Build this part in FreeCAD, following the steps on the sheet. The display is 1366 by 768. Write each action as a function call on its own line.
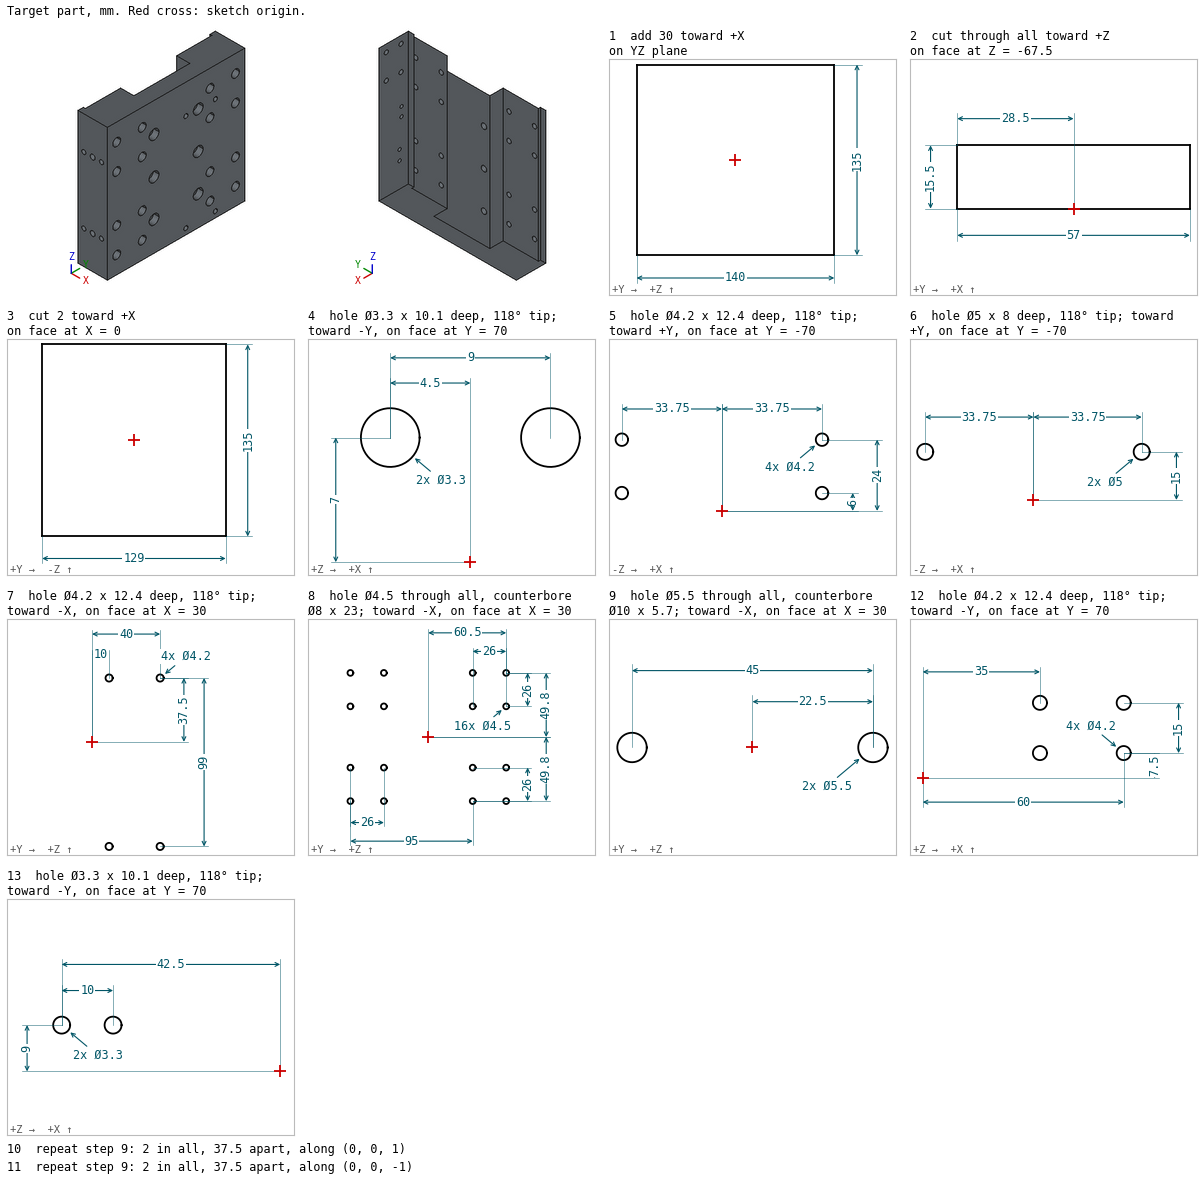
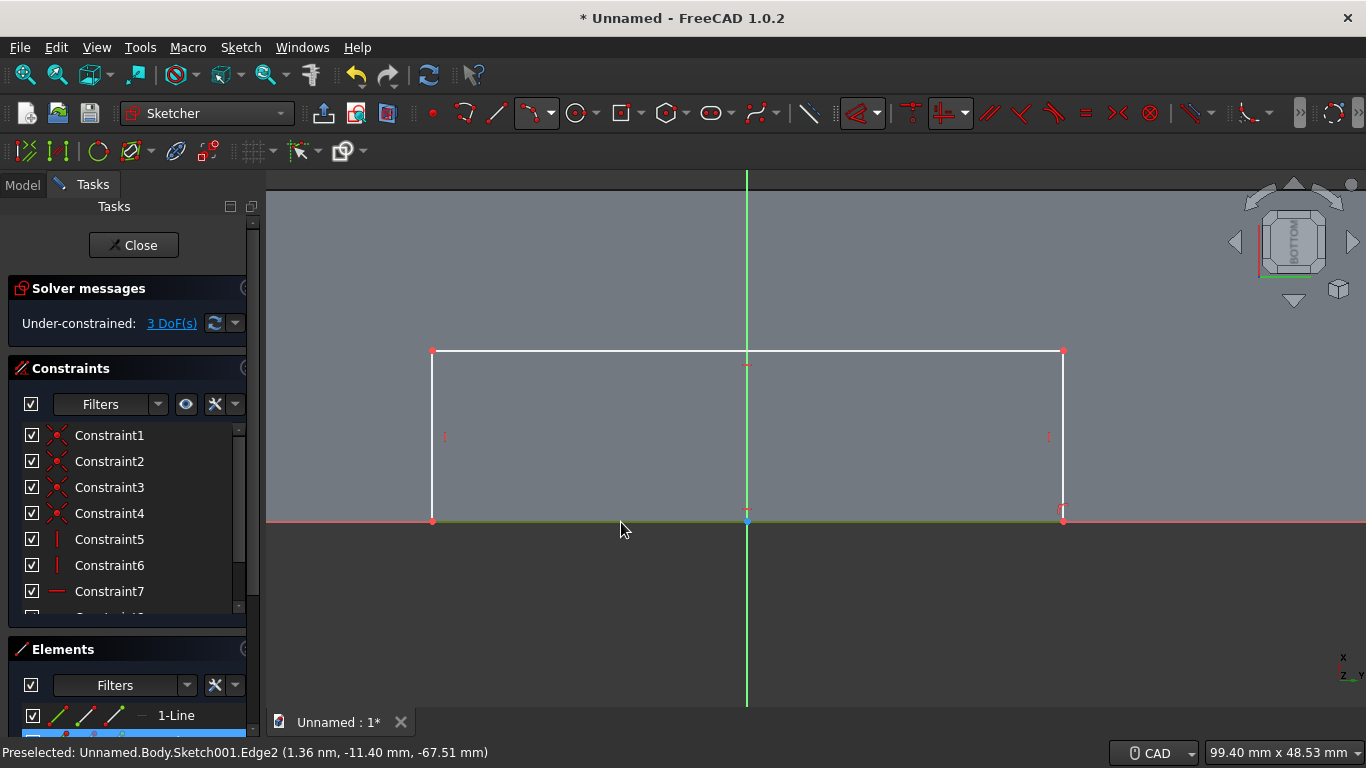
key(l)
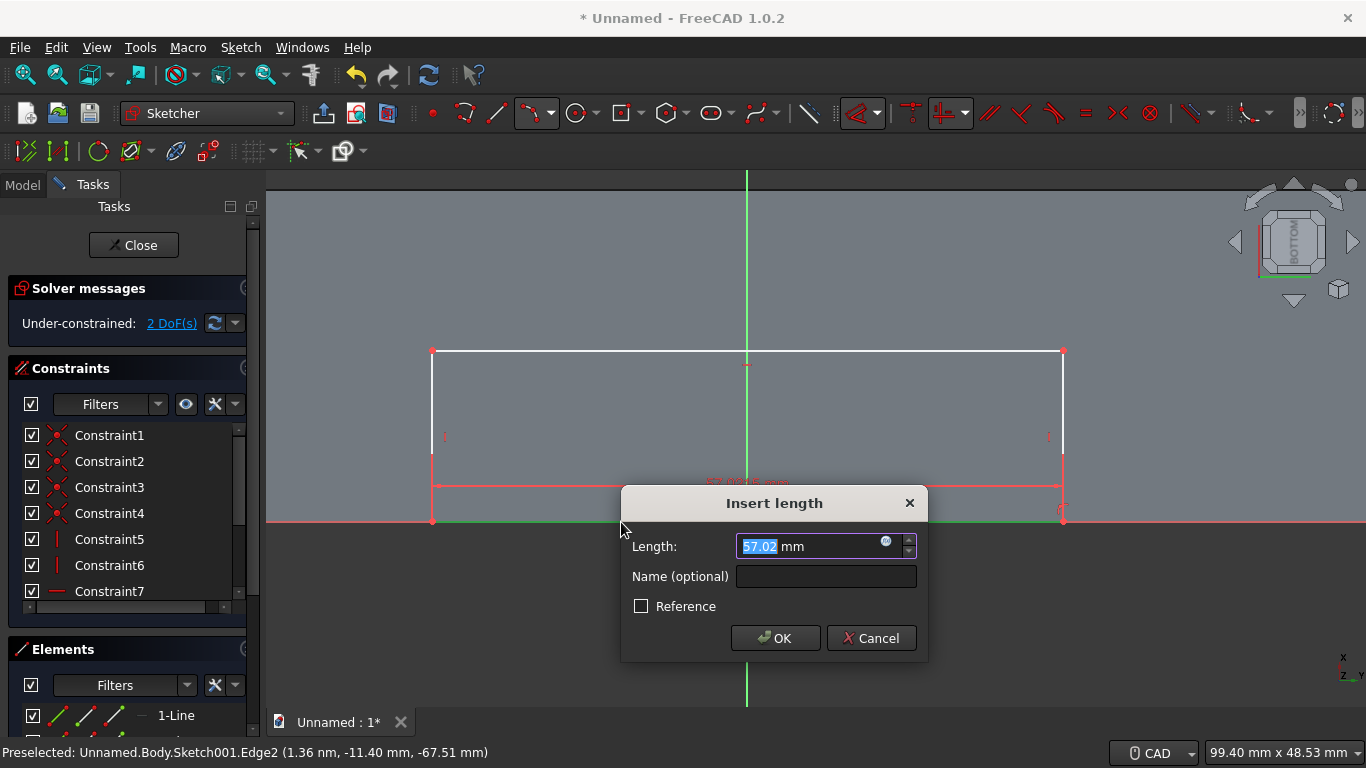
text(57)
key(Return)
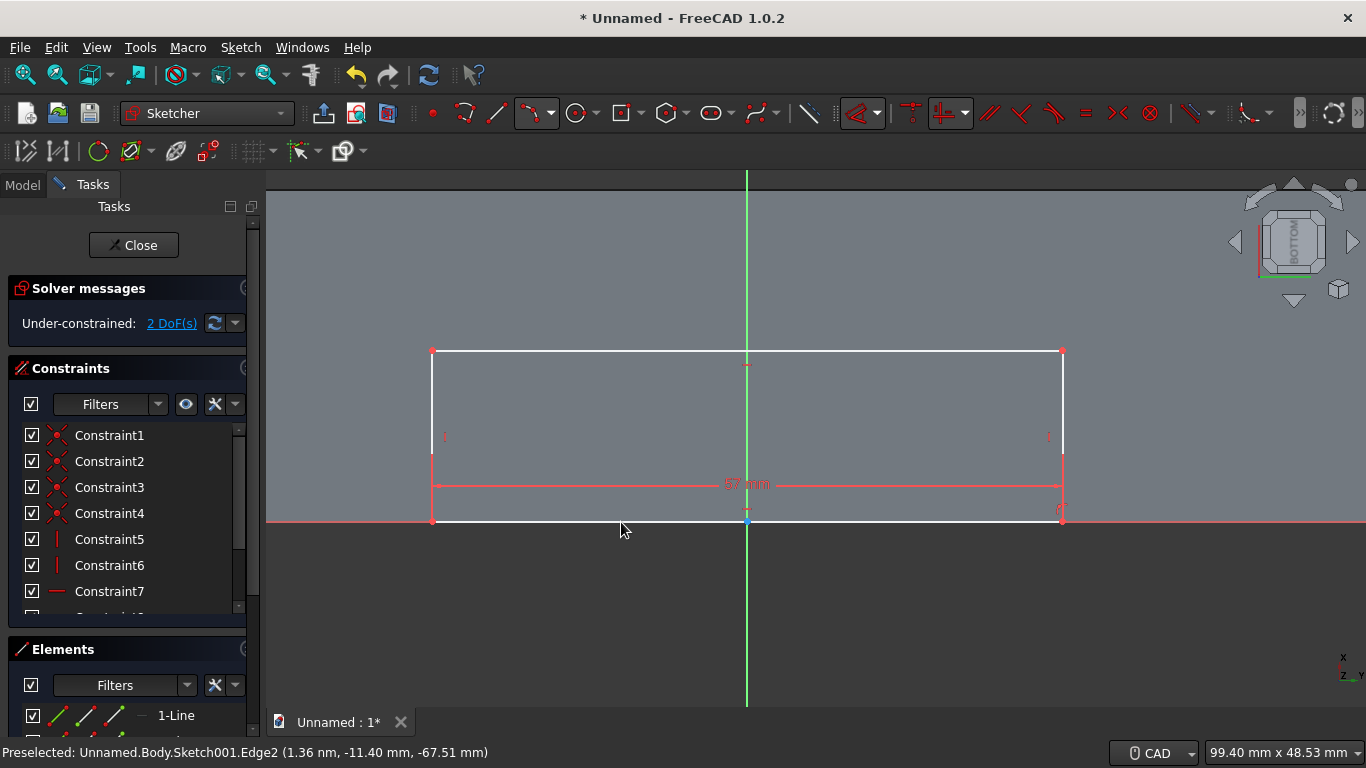
click(432, 402)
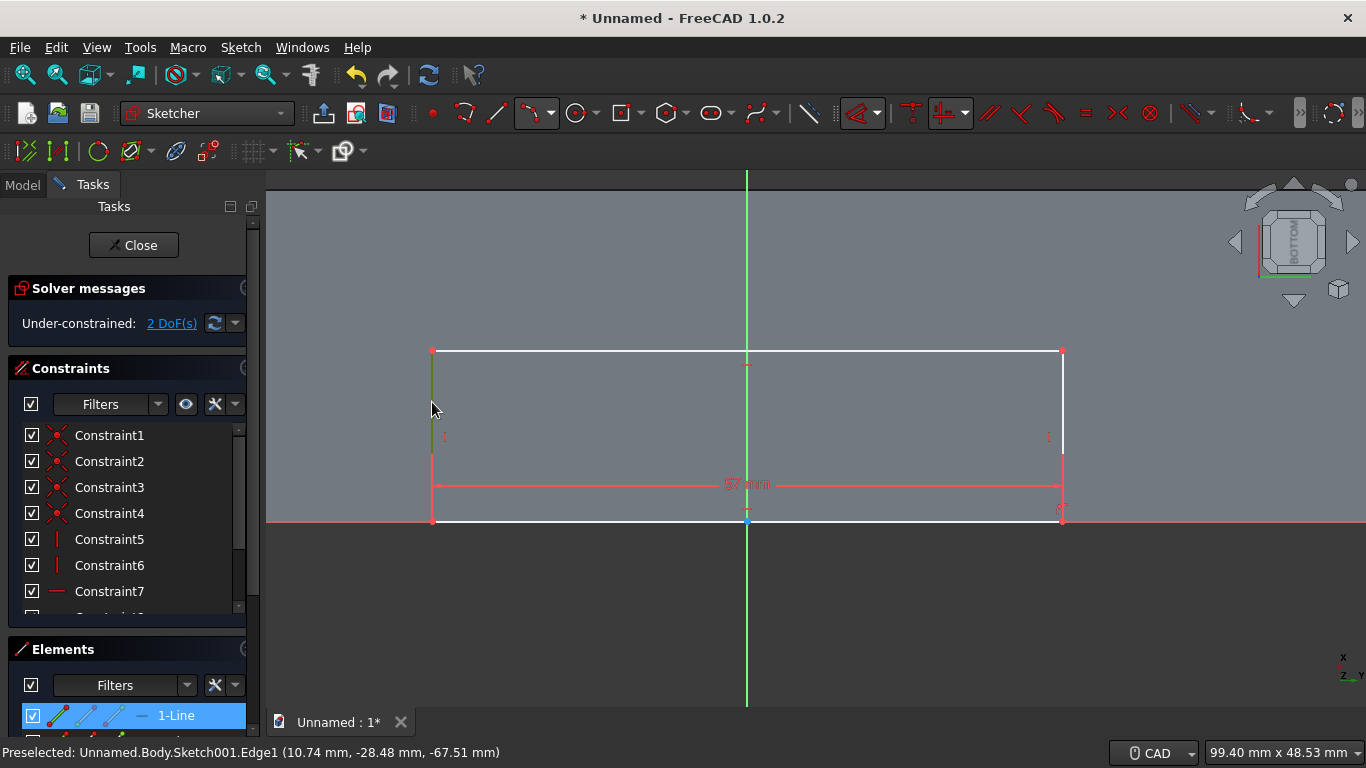
click(880, 114)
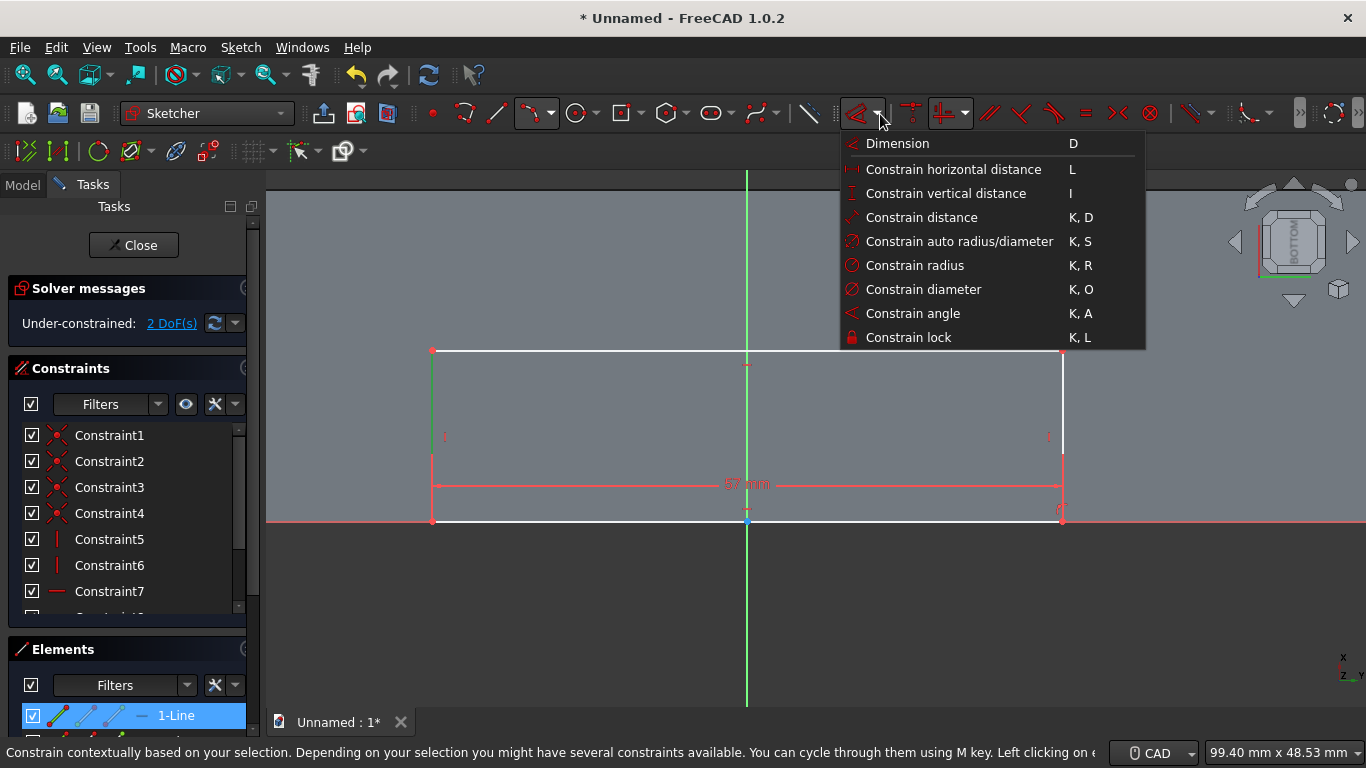
click(993, 193)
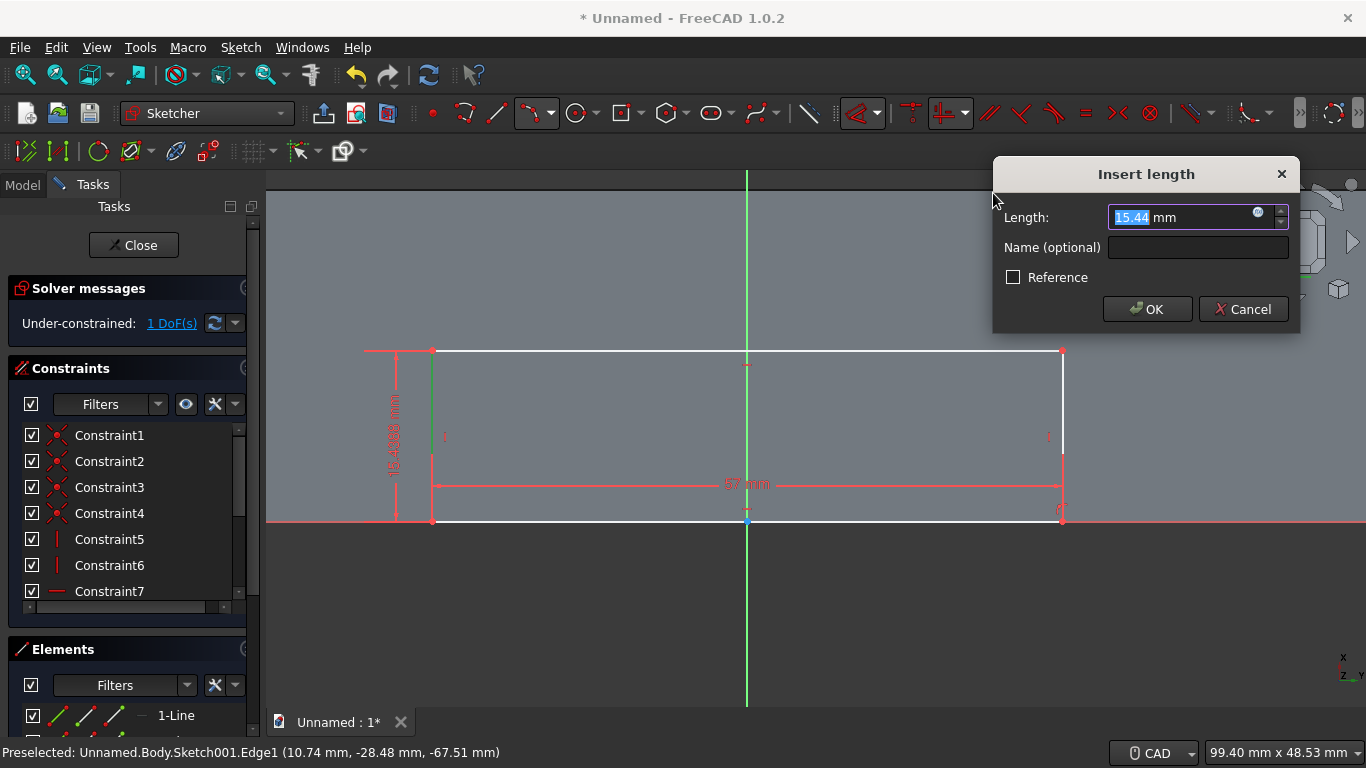
text(15.5)
key(Return)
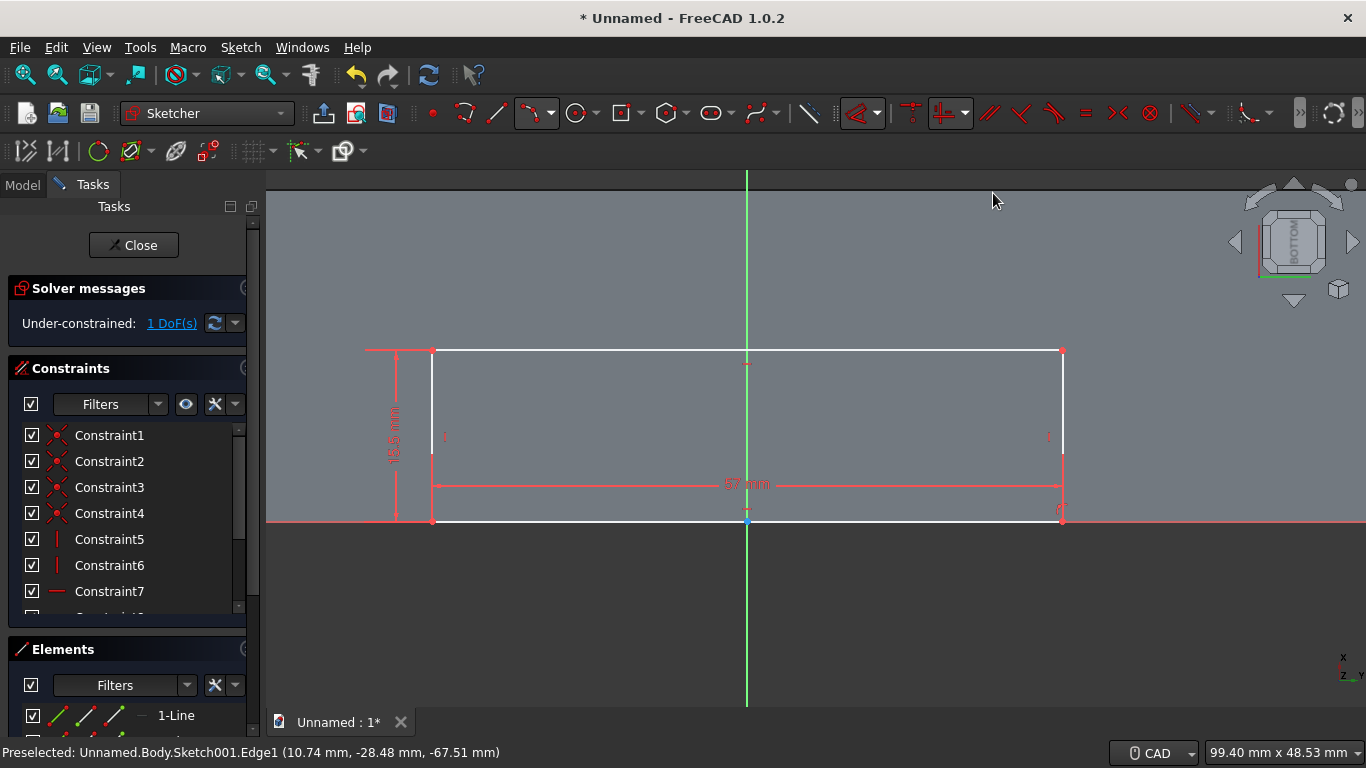
click(432, 350)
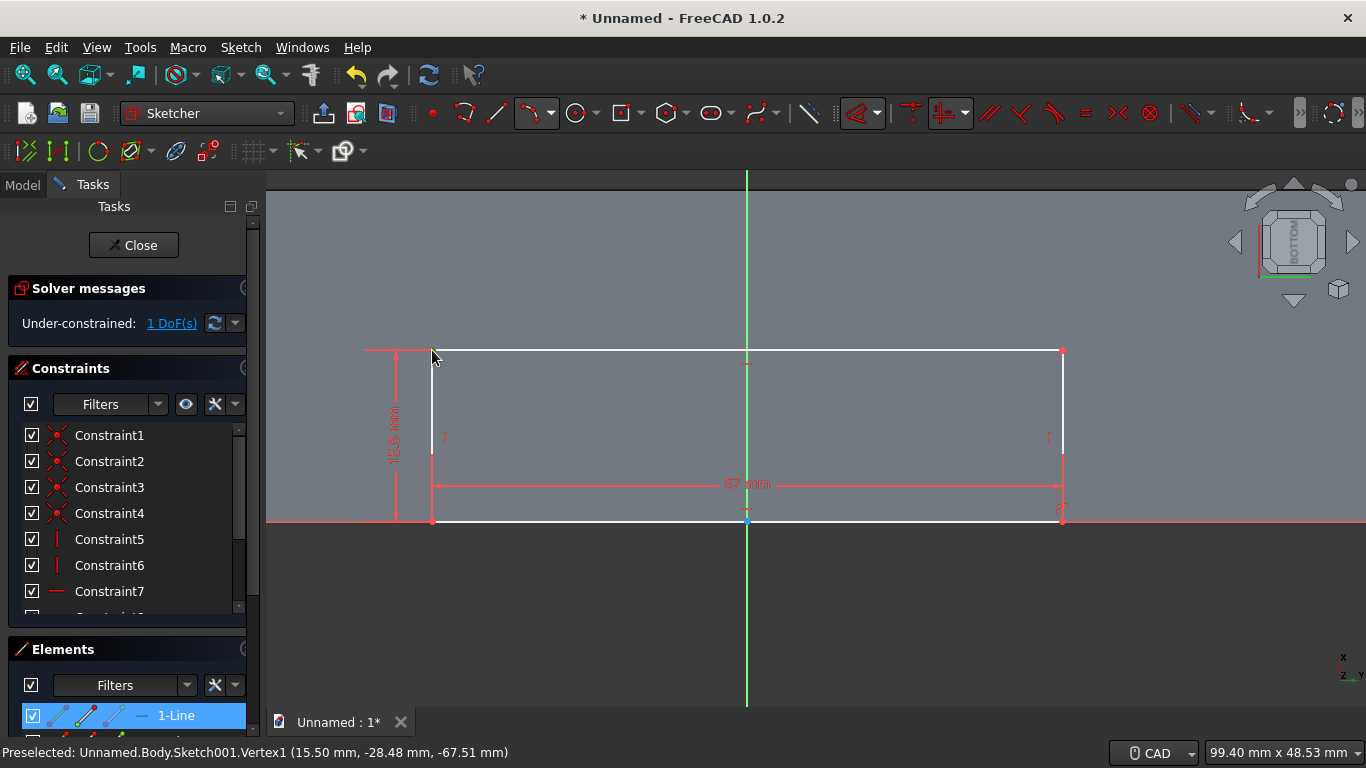
click(880, 114)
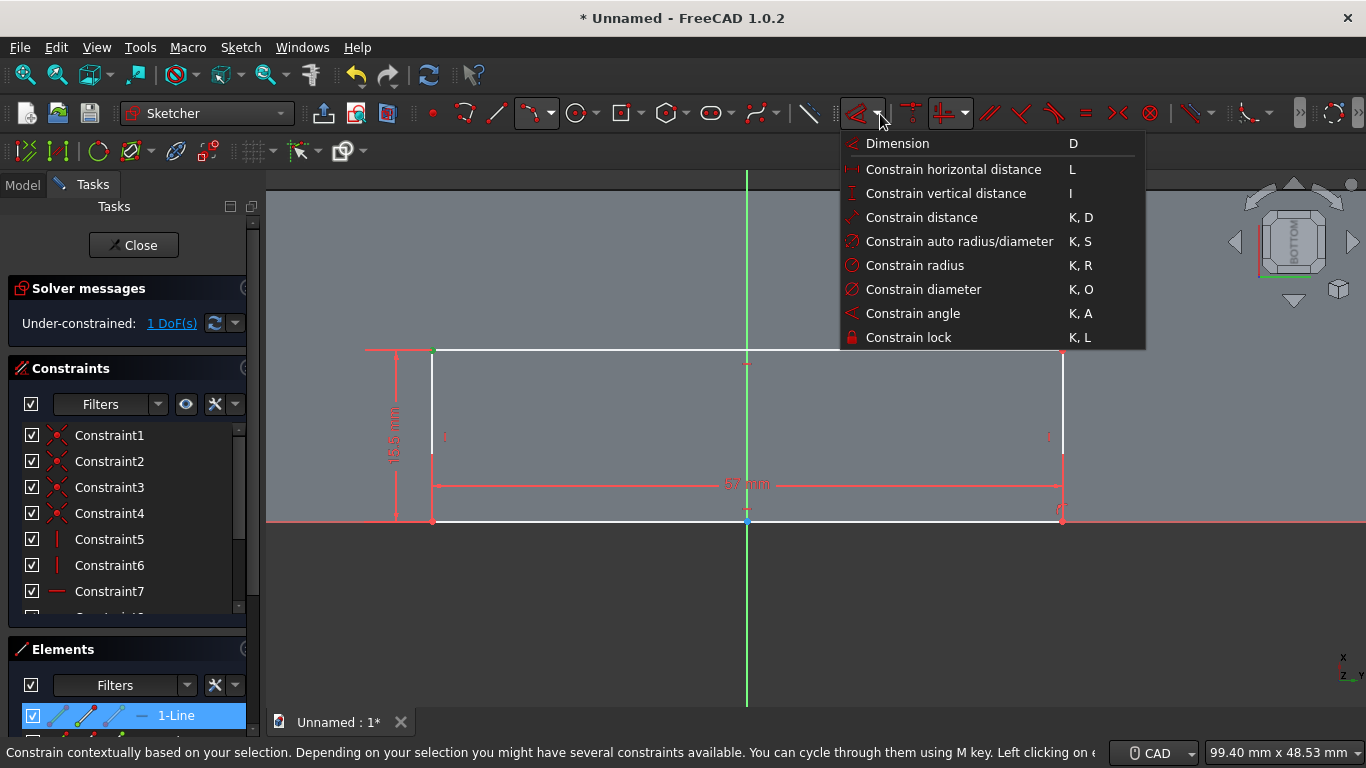
click(993, 169)